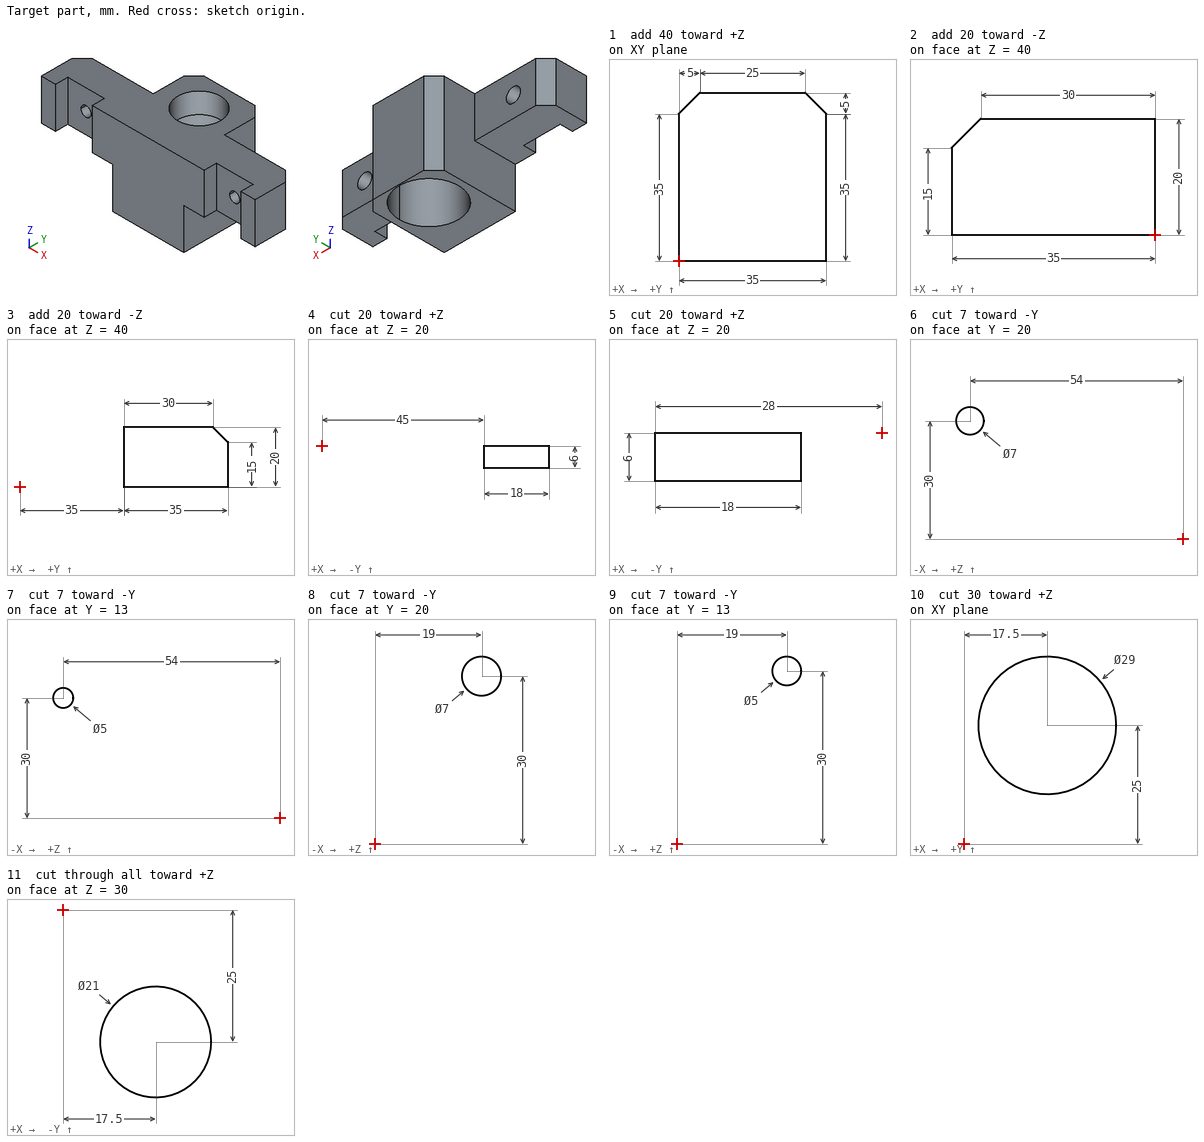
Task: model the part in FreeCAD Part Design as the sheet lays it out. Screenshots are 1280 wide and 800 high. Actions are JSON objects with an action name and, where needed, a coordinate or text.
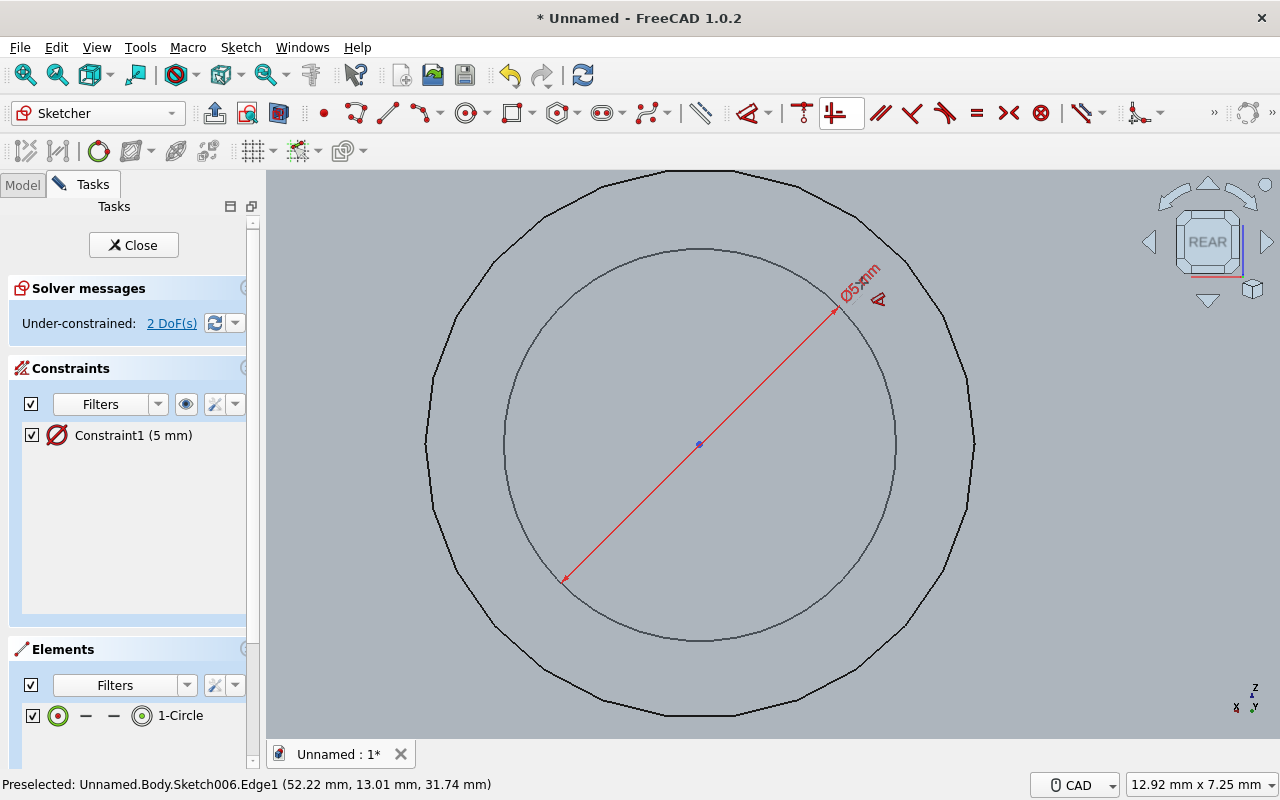
{"action": "left_click", "coordinate": [700, 445]}
{"action": "left_click", "coordinate": [907, 411]}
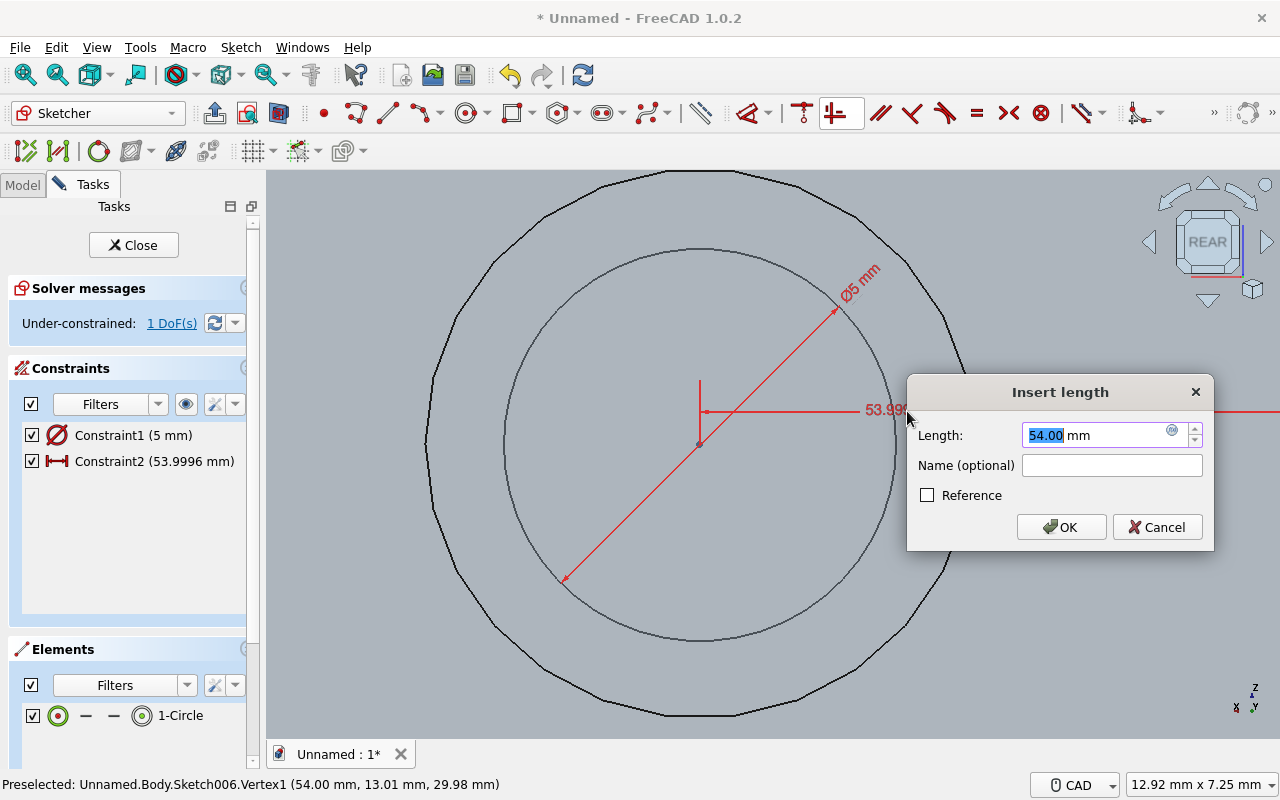
{"action": "type", "text": "54"}
{"action": "key", "text": "Return"}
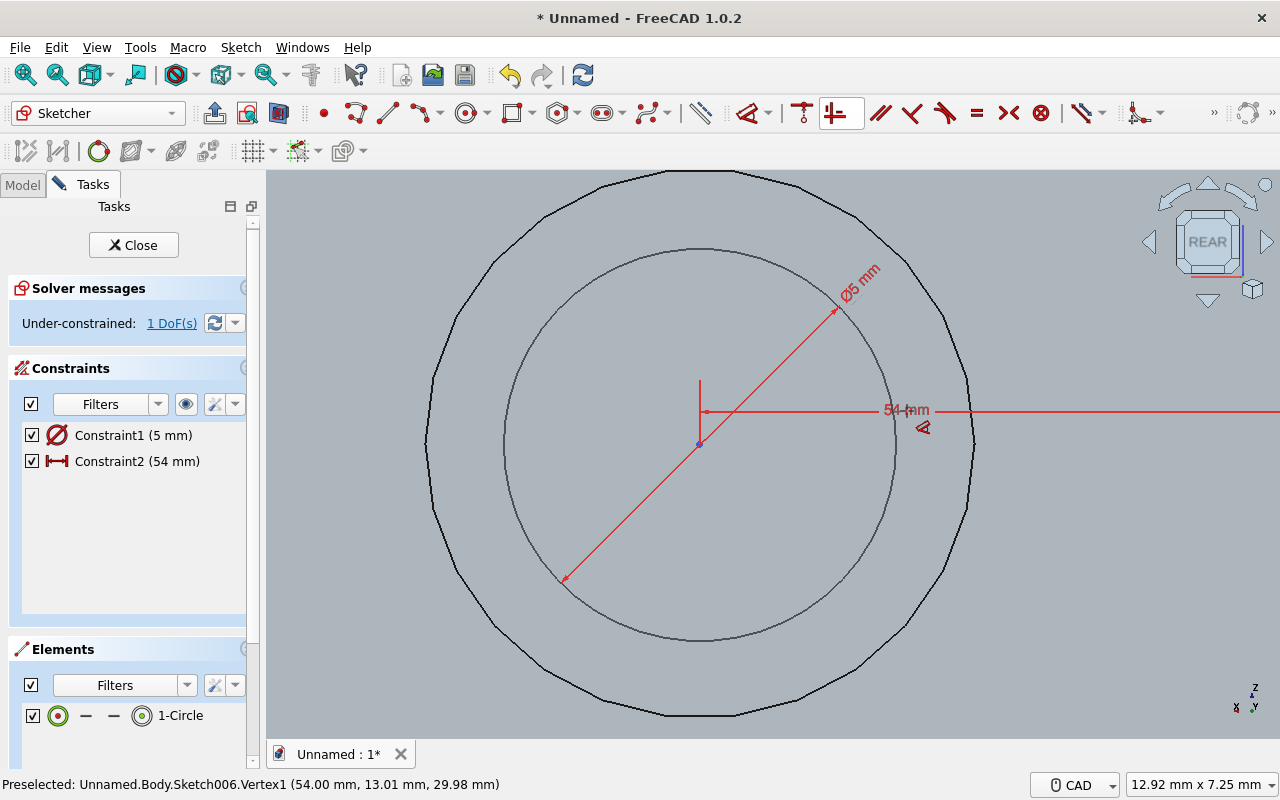
{"action": "left_click", "coordinate": [700, 445]}
{"action": "left_click", "coordinate": [666, 578]}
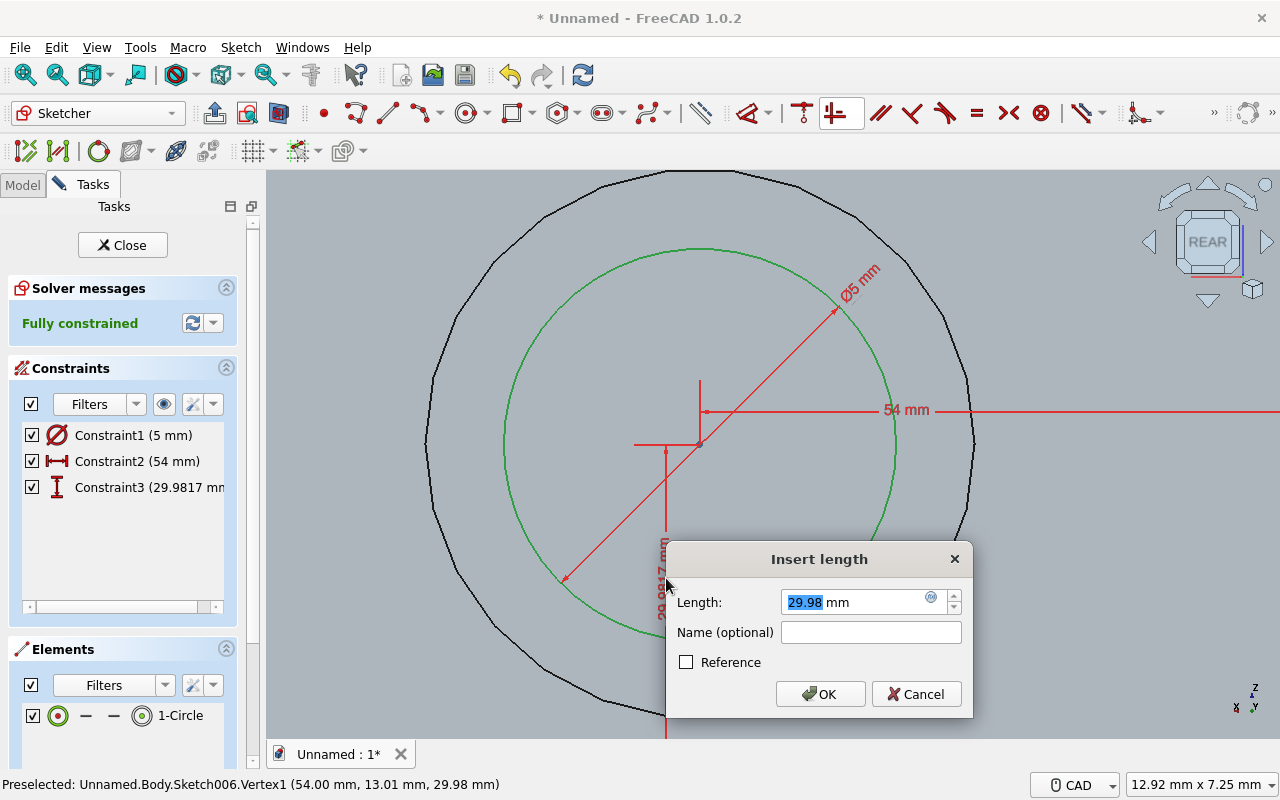
{"action": "type", "text": "30"}
{"action": "key", "text": "Return"}
{"action": "key", "text": "Escape"}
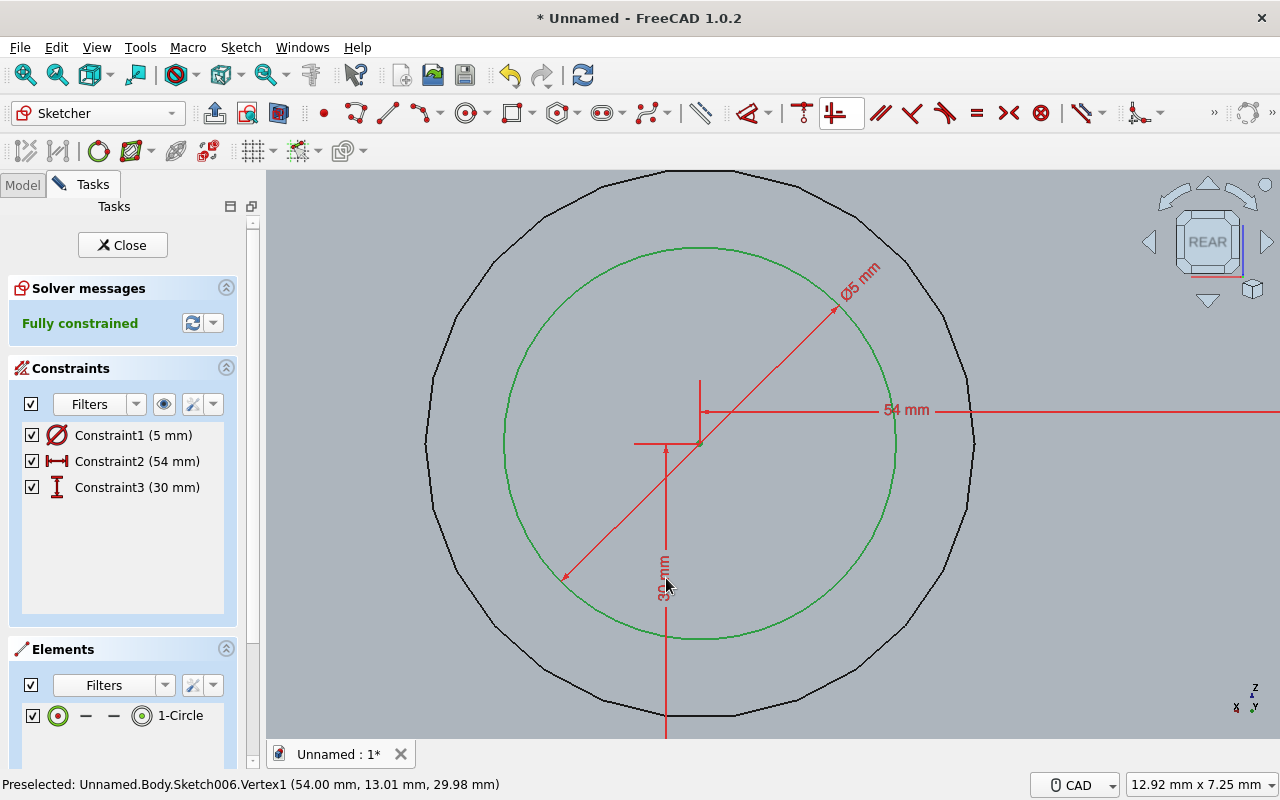
{"action": "left_click", "coordinate": [123, 245]}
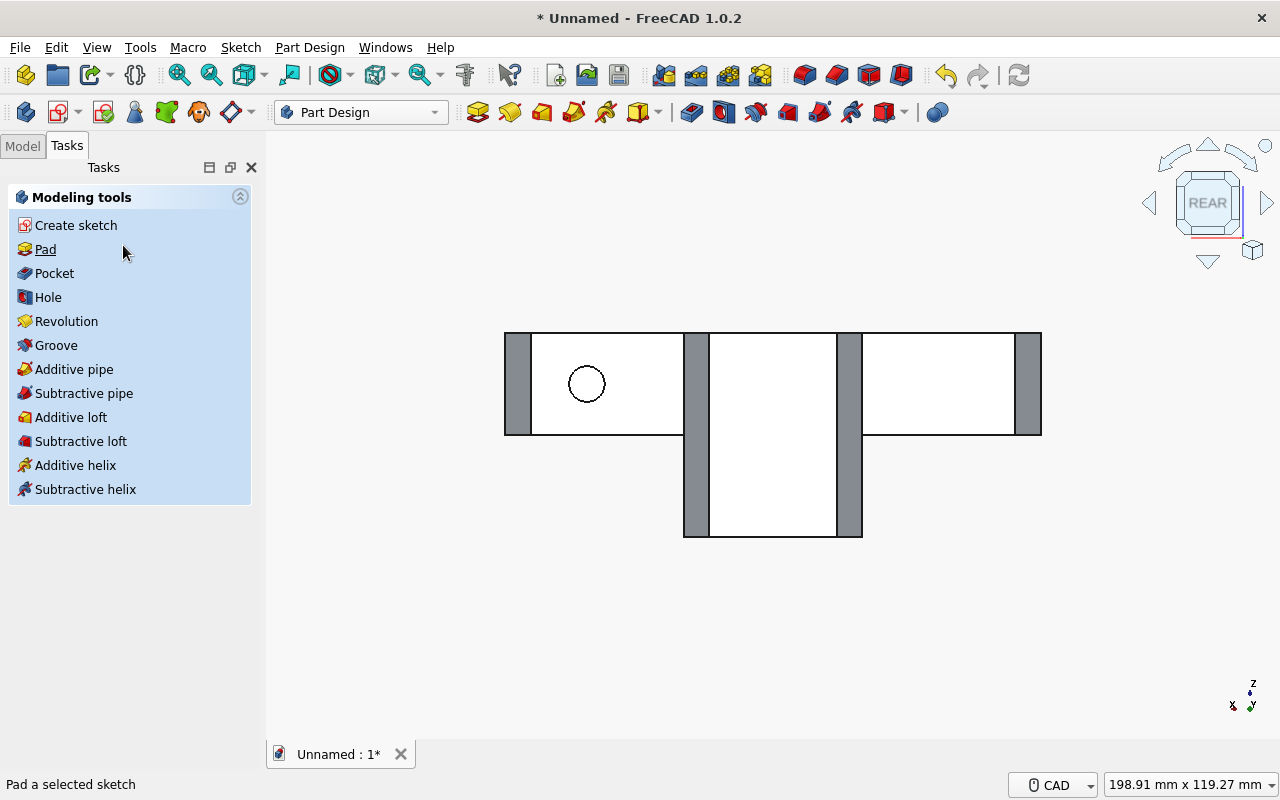
{"action": "left_click", "coordinate": [692, 112]}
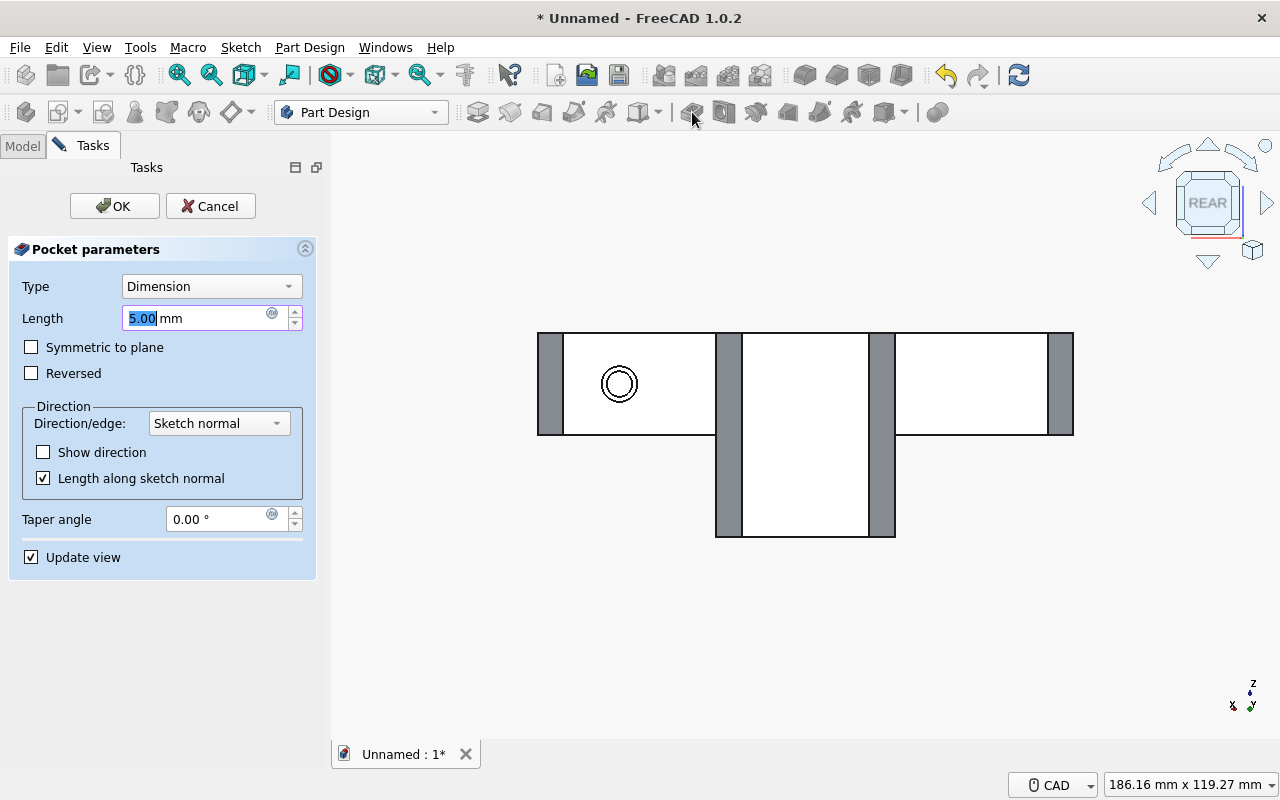
{"action": "type", "text": "7"}
{"action": "key", "text": "Tab"}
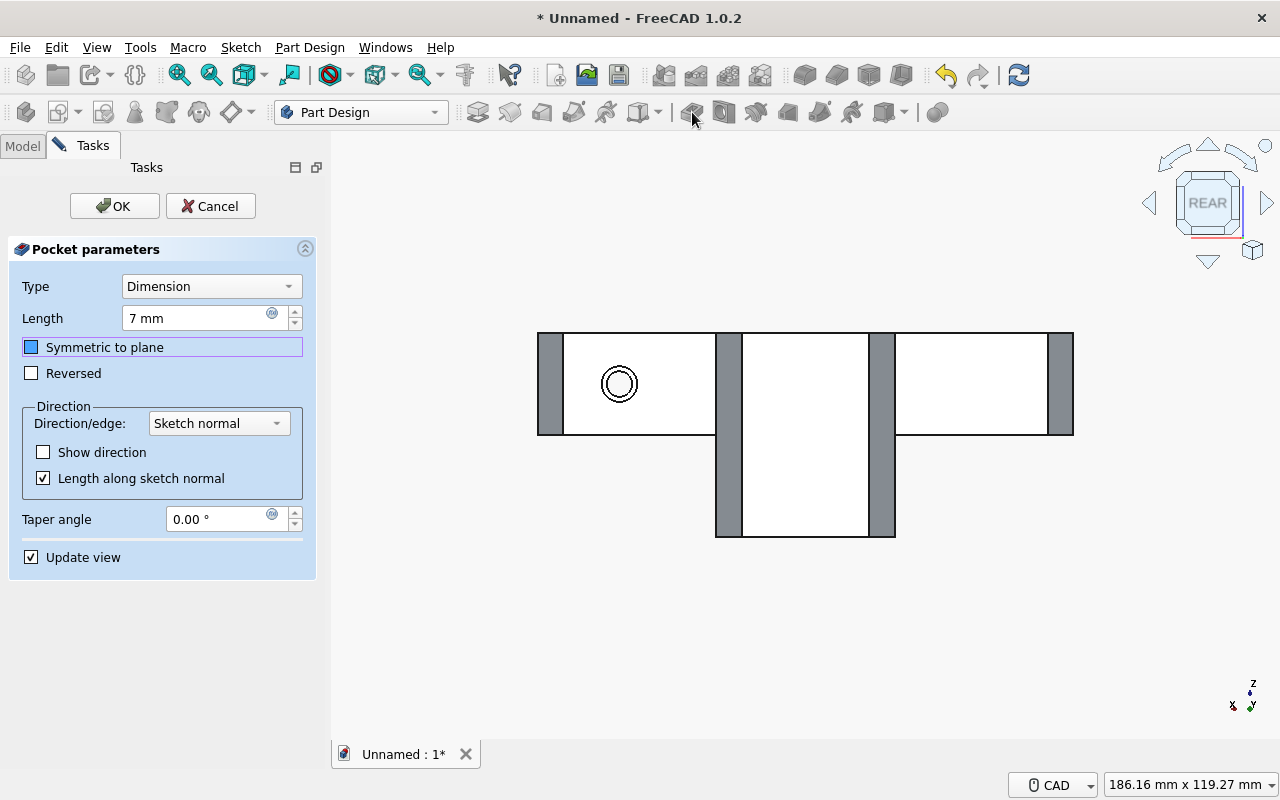
{"action": "left_click", "coordinate": [115, 206]}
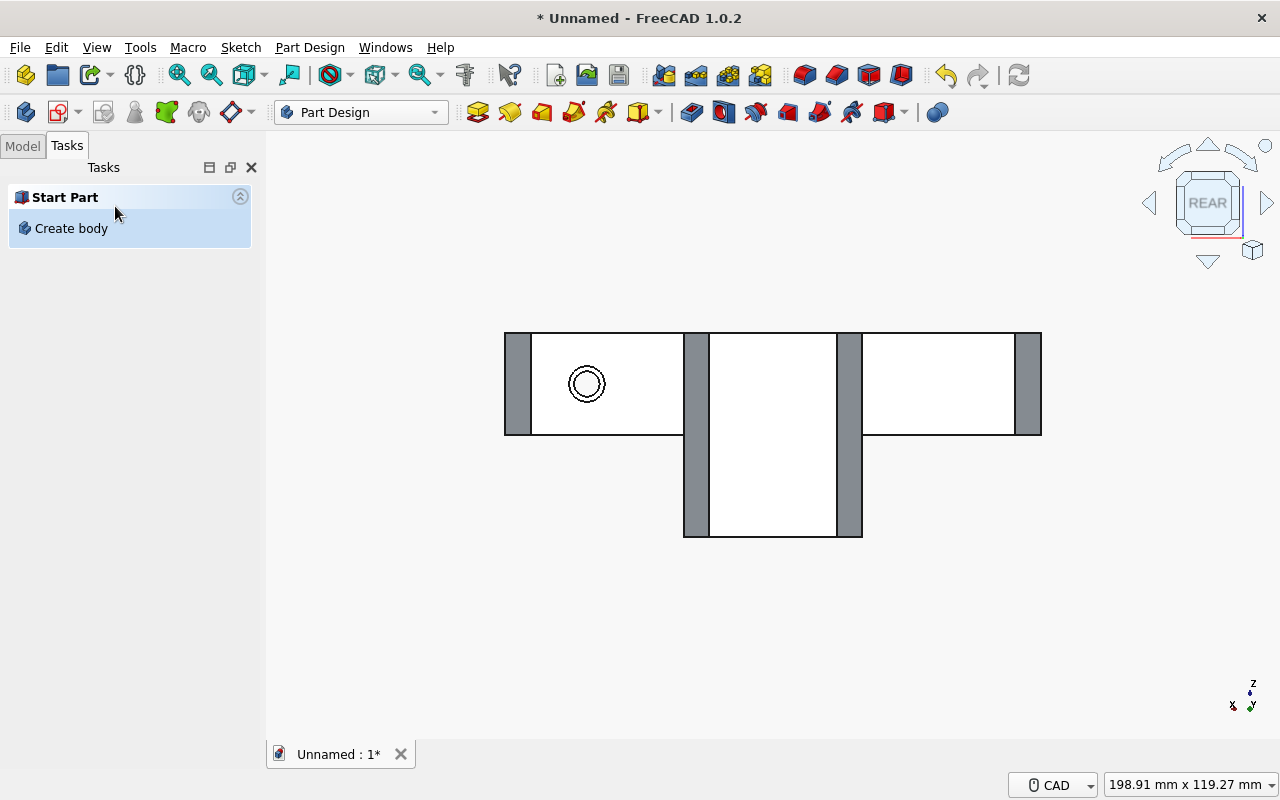
{"action": "left_click", "coordinate": [917, 383]}